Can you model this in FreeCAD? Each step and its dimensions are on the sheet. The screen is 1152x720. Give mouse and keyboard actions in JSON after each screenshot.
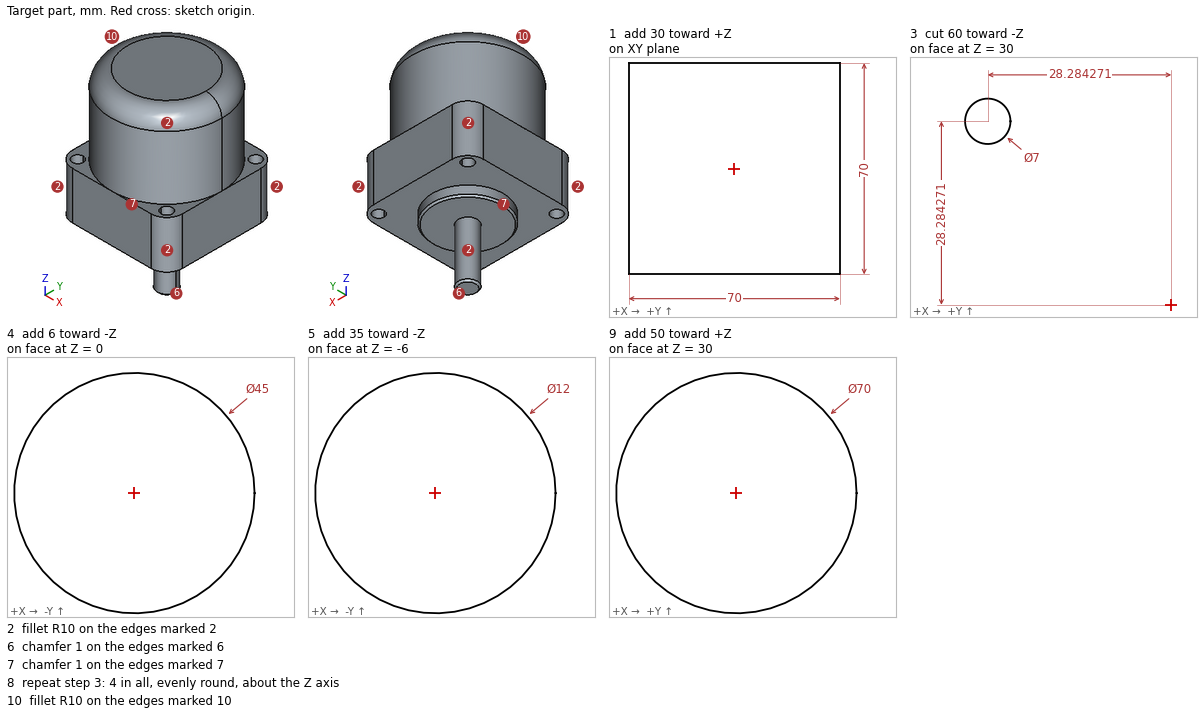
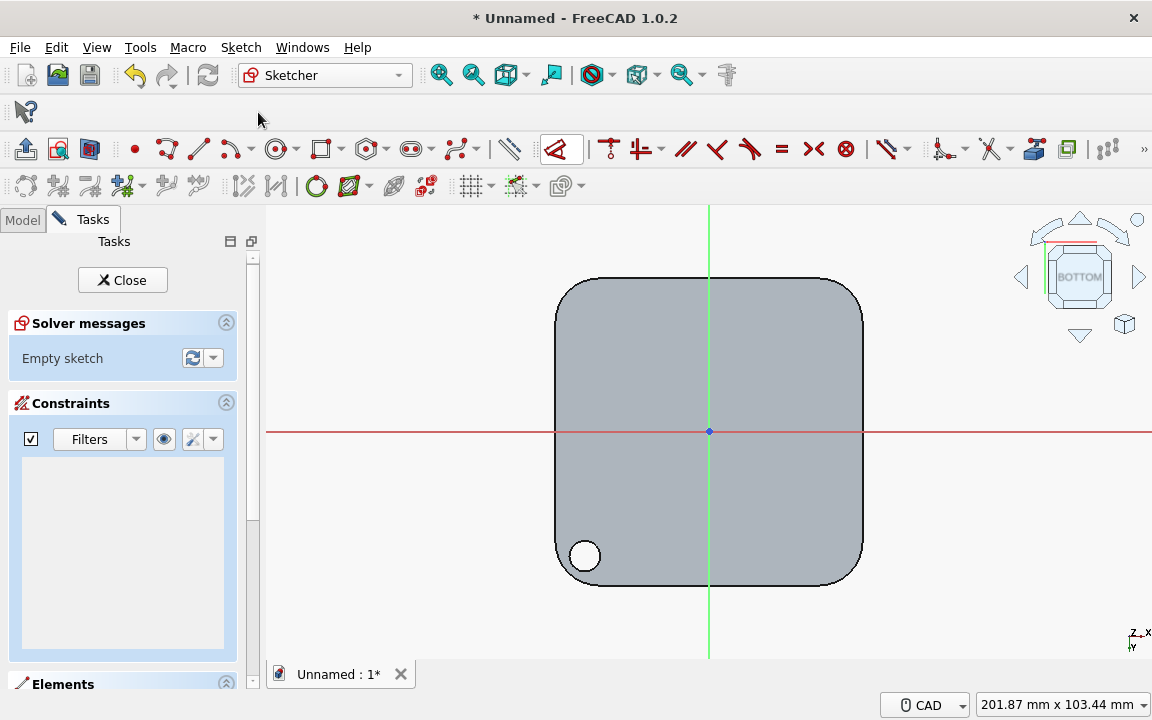
{"action": "scroll", "coordinate": [848, 432], "scroll_direction": "up", "scroll_amount": 2}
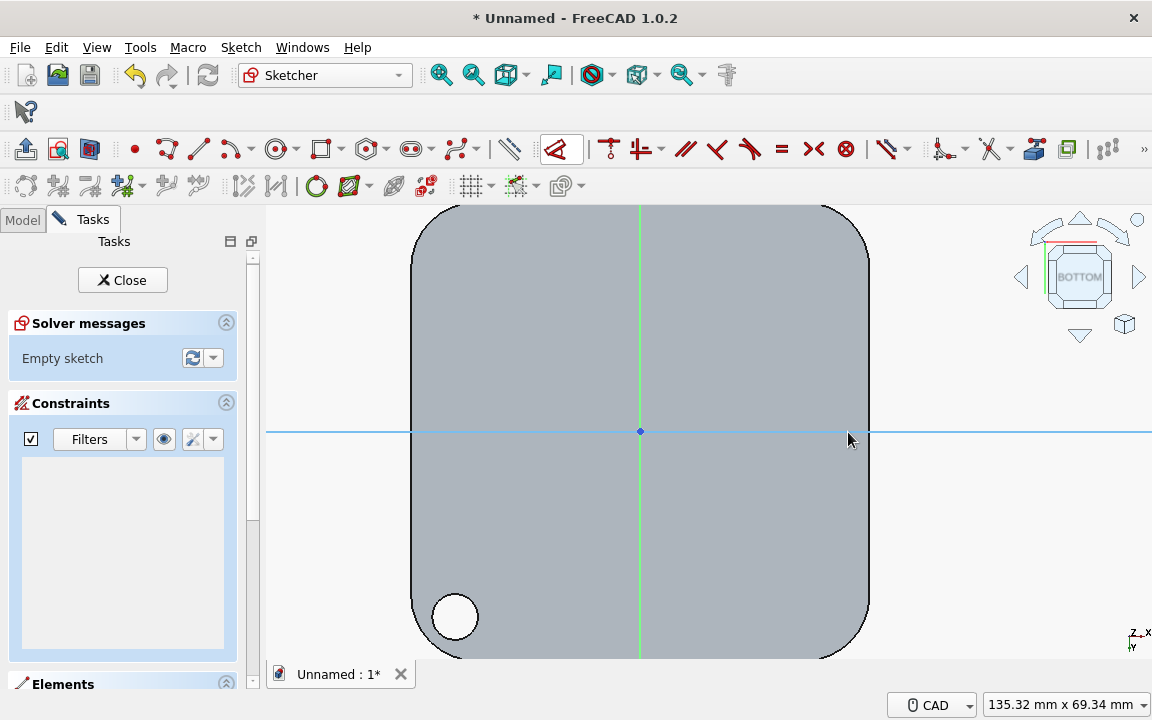
{"action": "key", "text": "g c"}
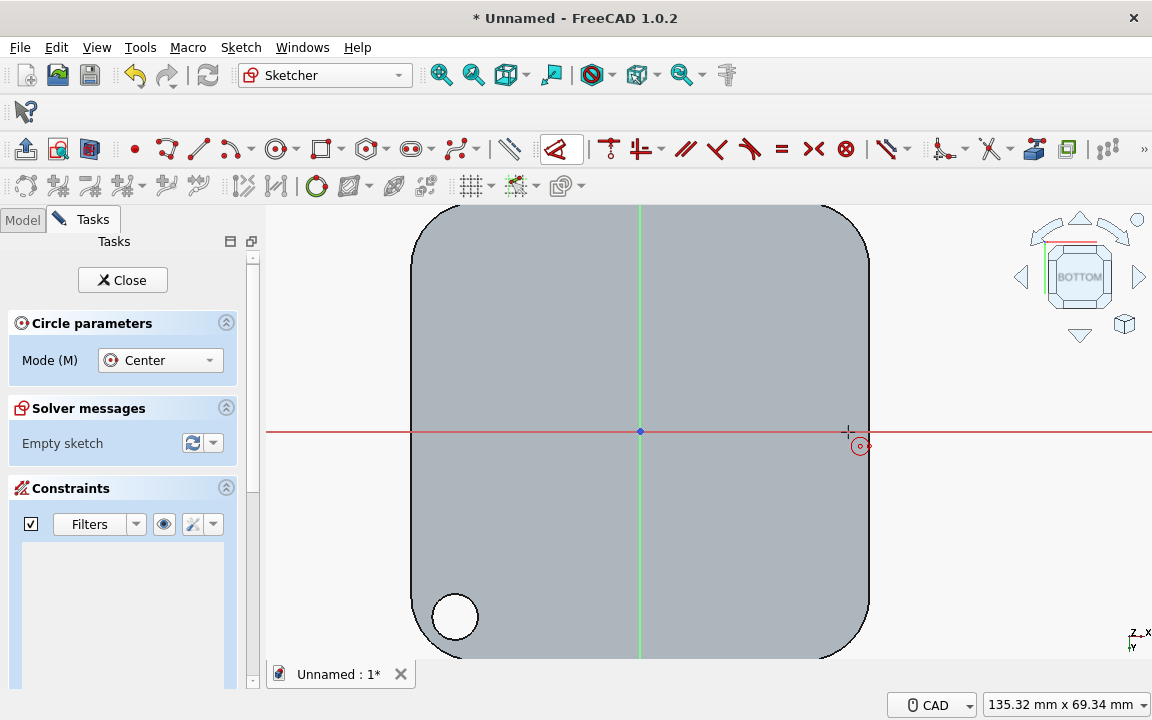
{"action": "left_click", "coordinate": [640, 432]}
{"action": "mouse_move", "coordinate": [744, 328]}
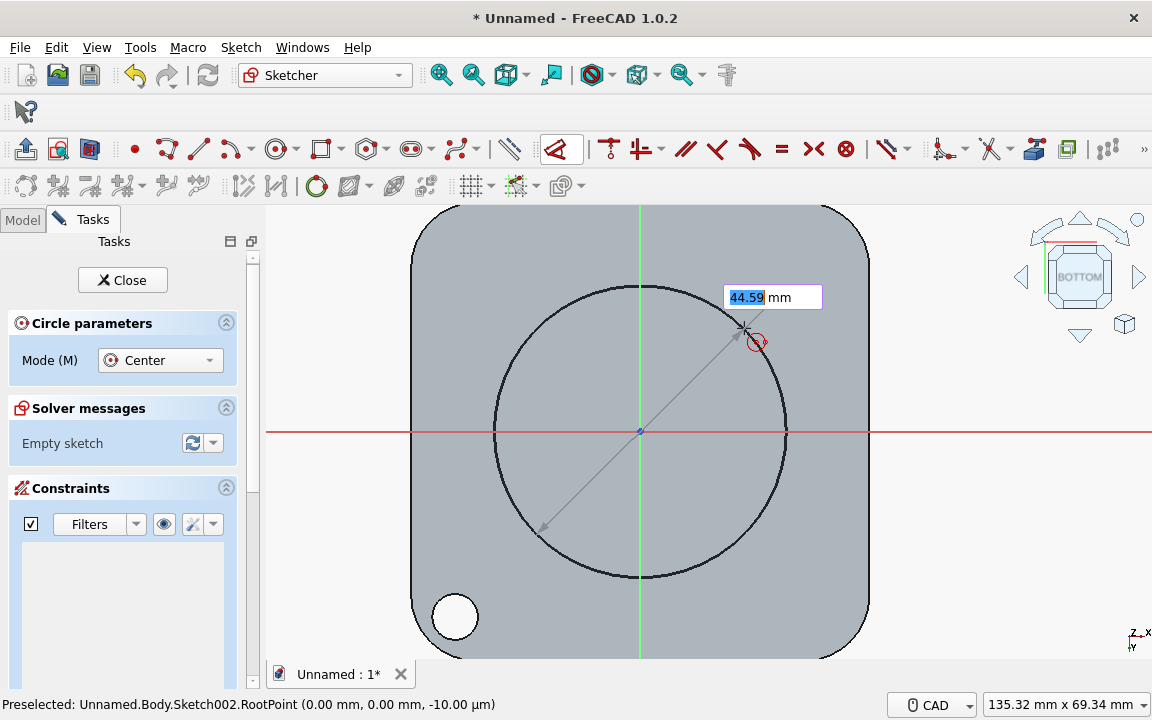
{"action": "type", "text": "45"}
{"action": "key", "text": "Return"}
{"action": "key", "text": "Escape"}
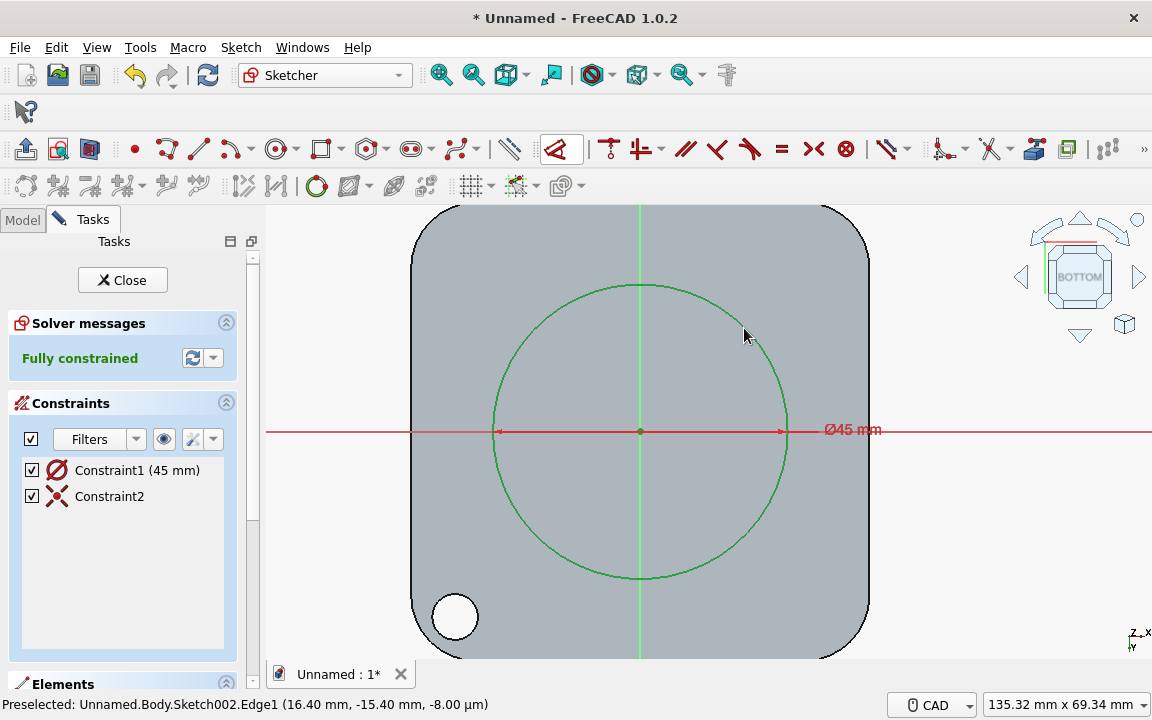
{"action": "left_click", "coordinate": [123, 280]}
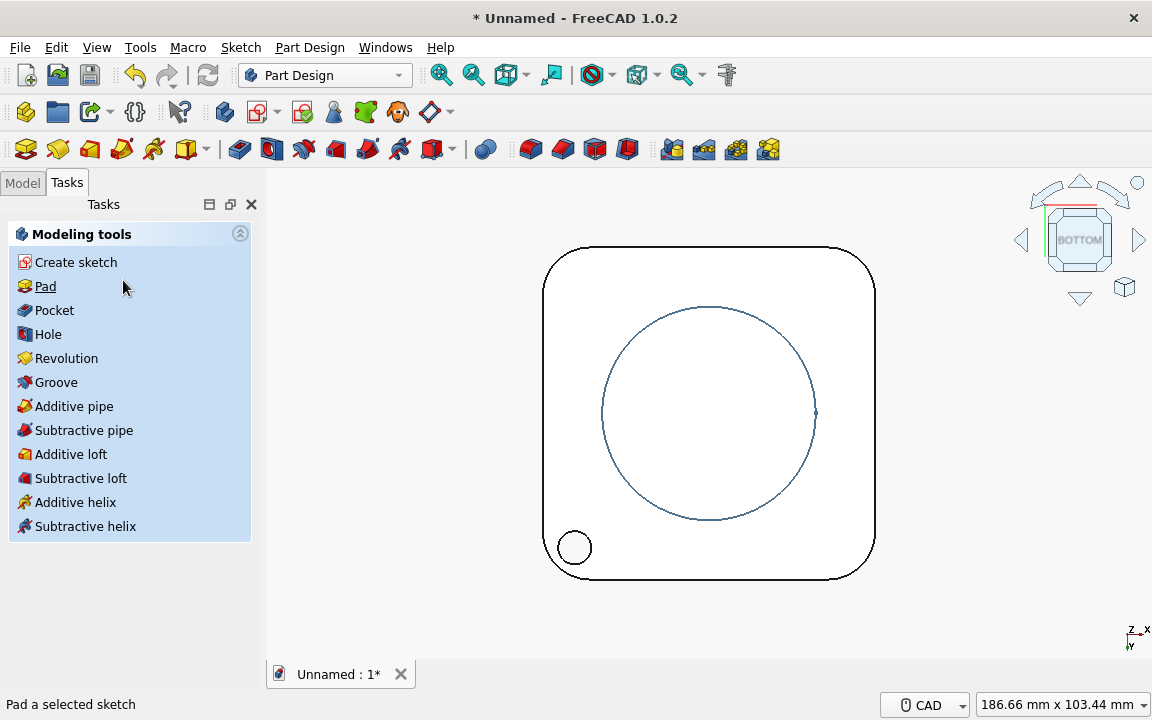
{"action": "left_click", "coordinate": [26, 150]}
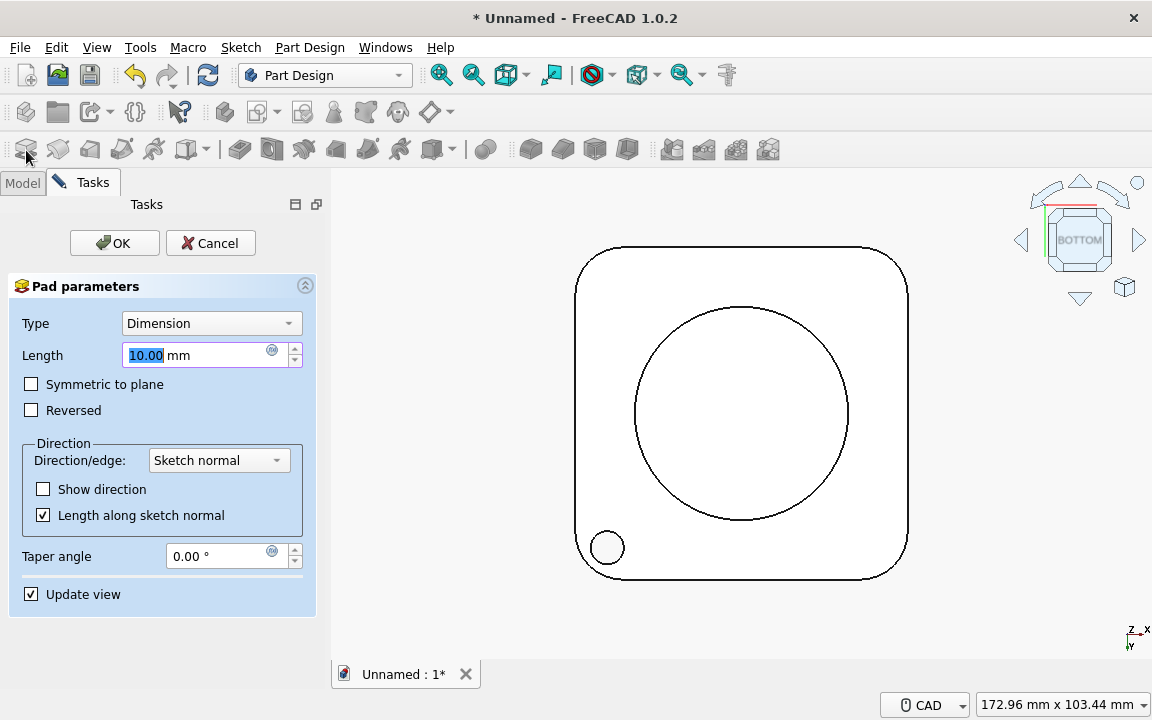
{"action": "type", "text": "6"}
{"action": "key", "text": "Tab"}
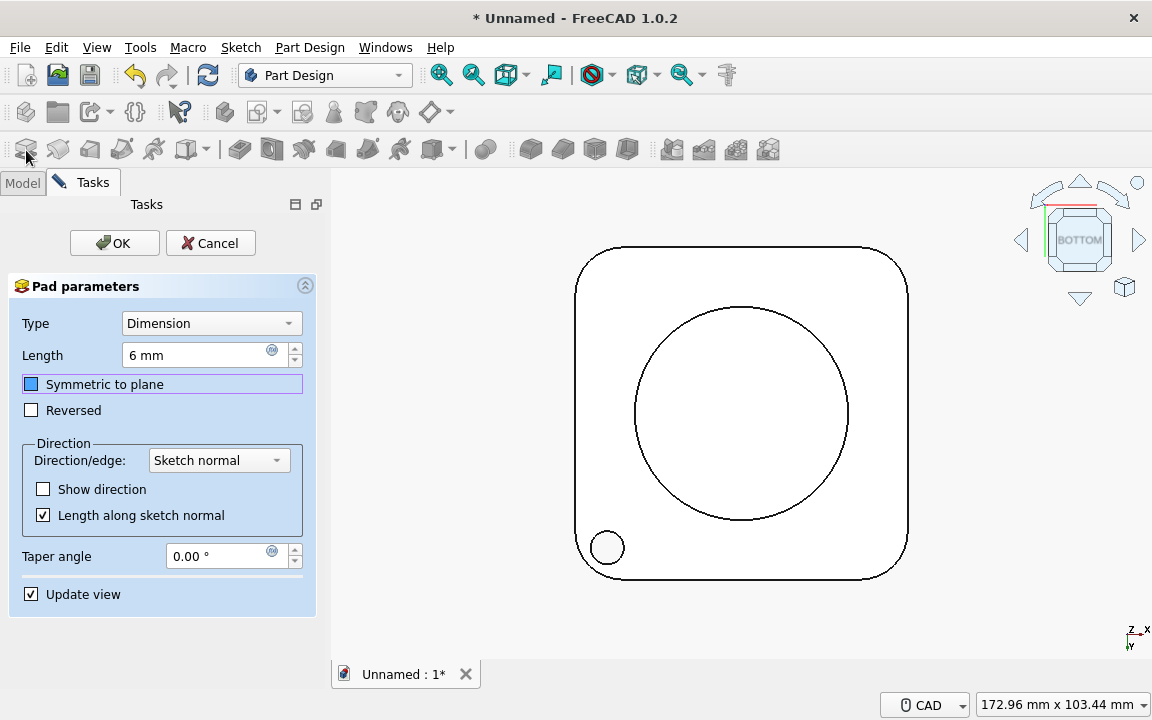
{"action": "left_click", "coordinate": [115, 243]}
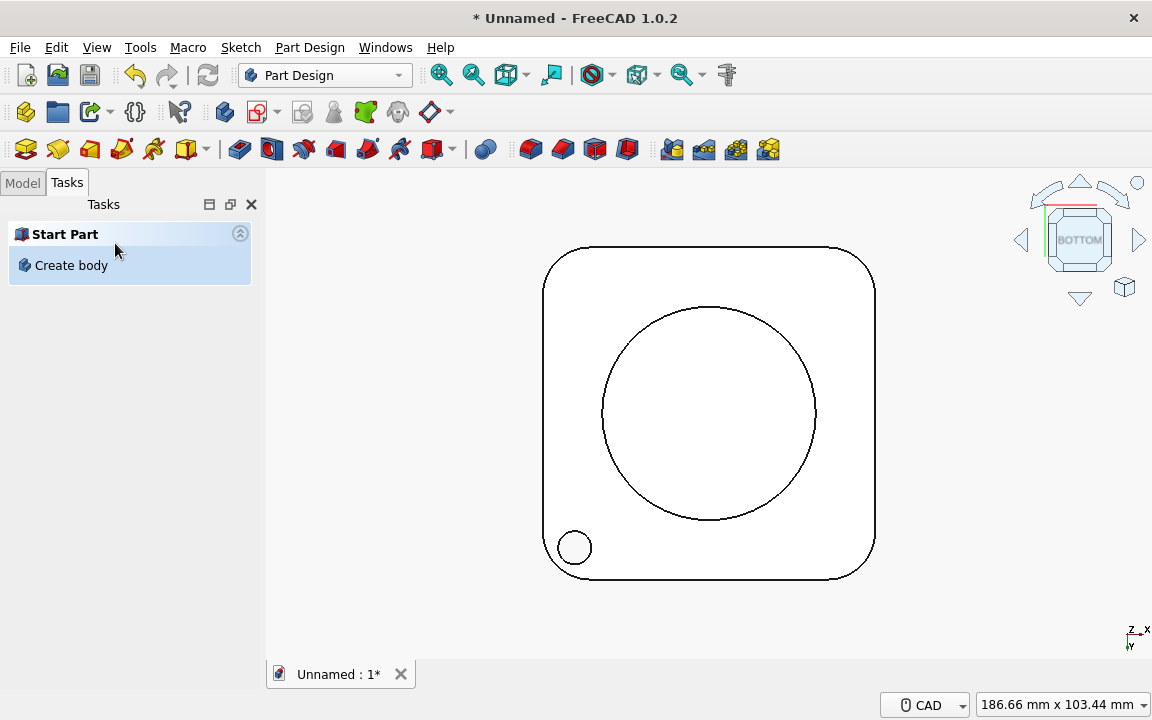
{"action": "left_click", "coordinate": [709, 413]}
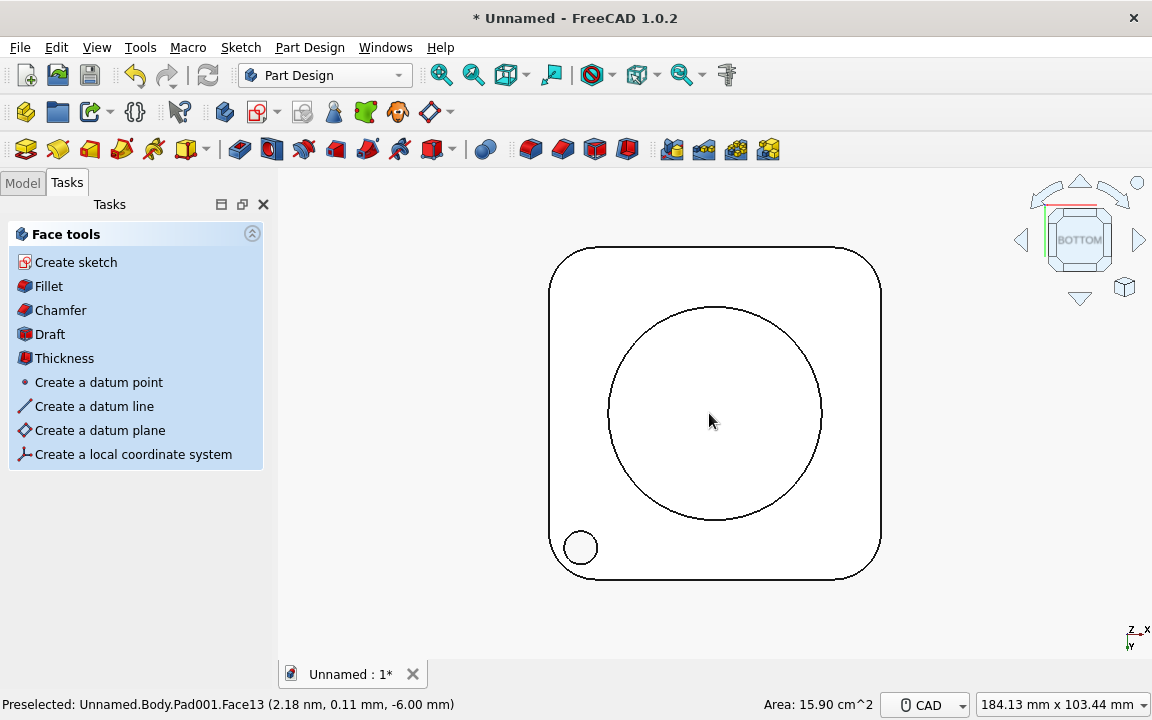
{"action": "left_click", "coordinate": [258, 112]}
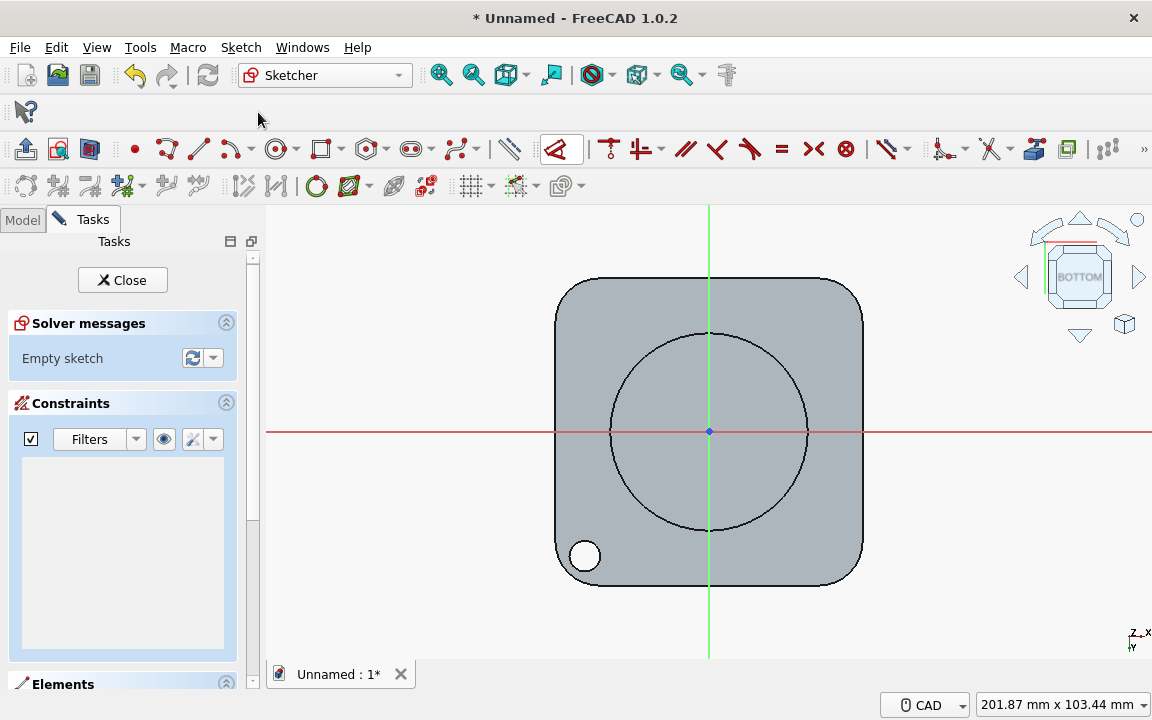
{"action": "scroll", "coordinate": [726, 432], "scroll_direction": "up", "scroll_amount": 8}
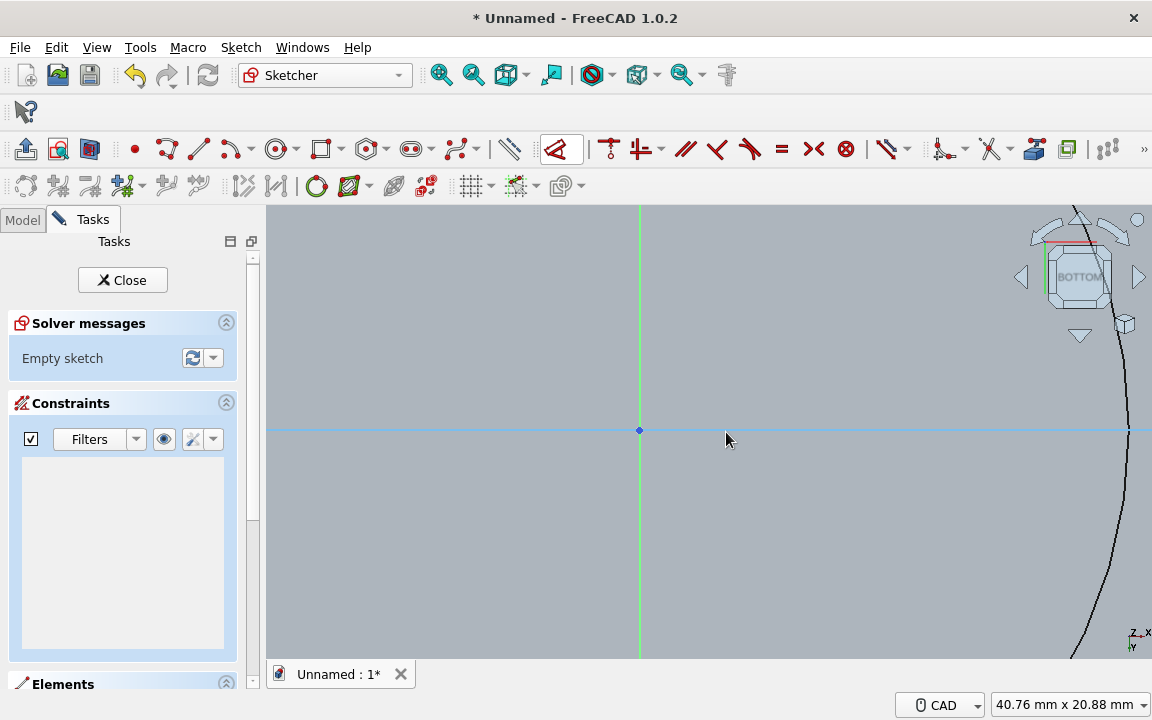
{"action": "left_click", "coordinate": [276, 150]}